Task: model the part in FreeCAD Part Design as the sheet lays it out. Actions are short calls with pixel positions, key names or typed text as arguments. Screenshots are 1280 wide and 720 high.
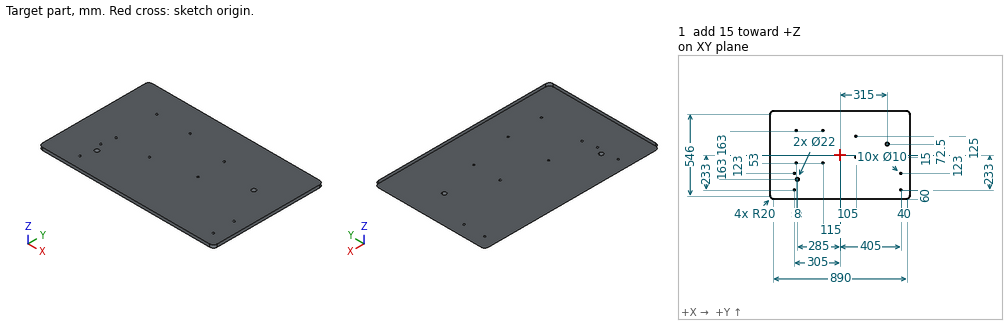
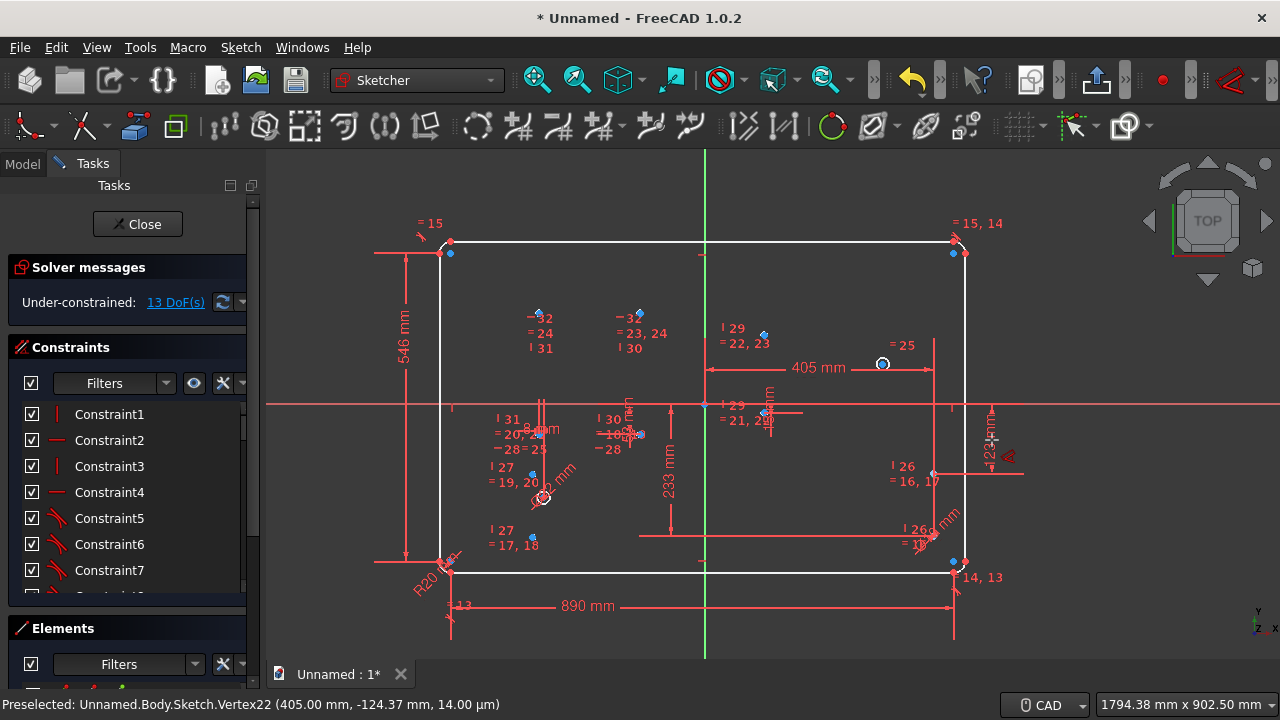
click(533, 537)
click(619, 370)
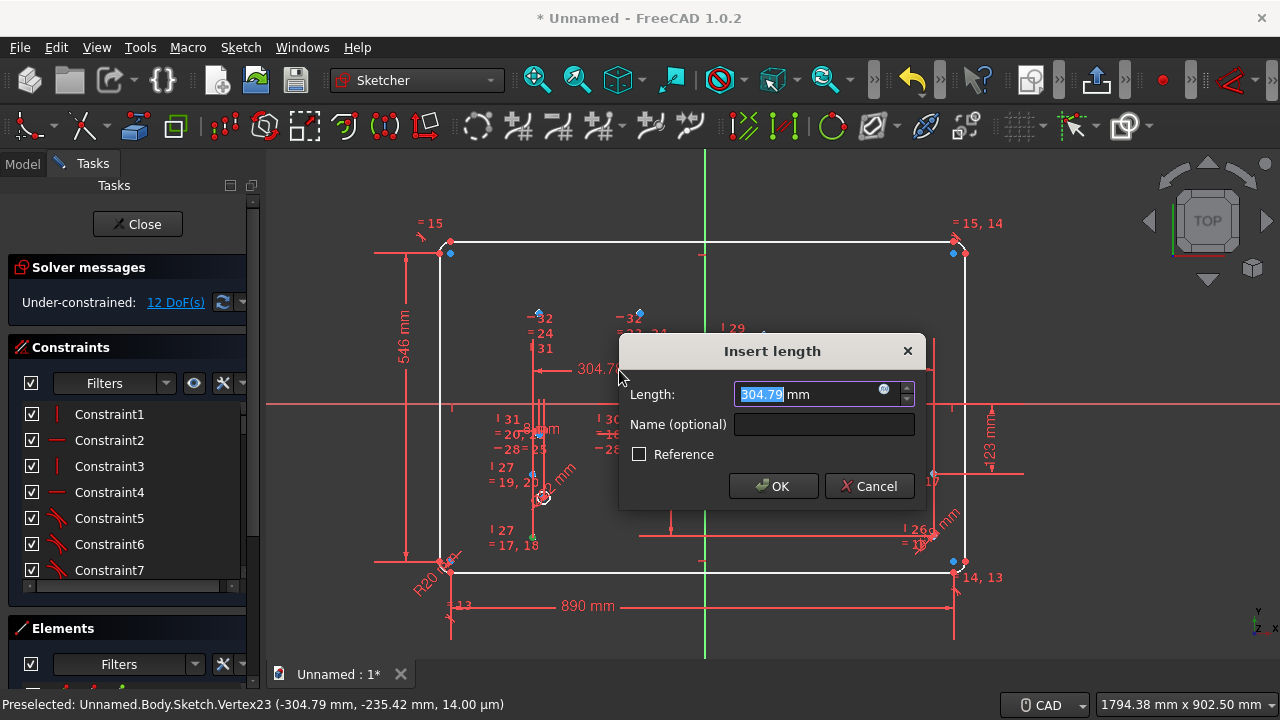
text(305)
key(Return)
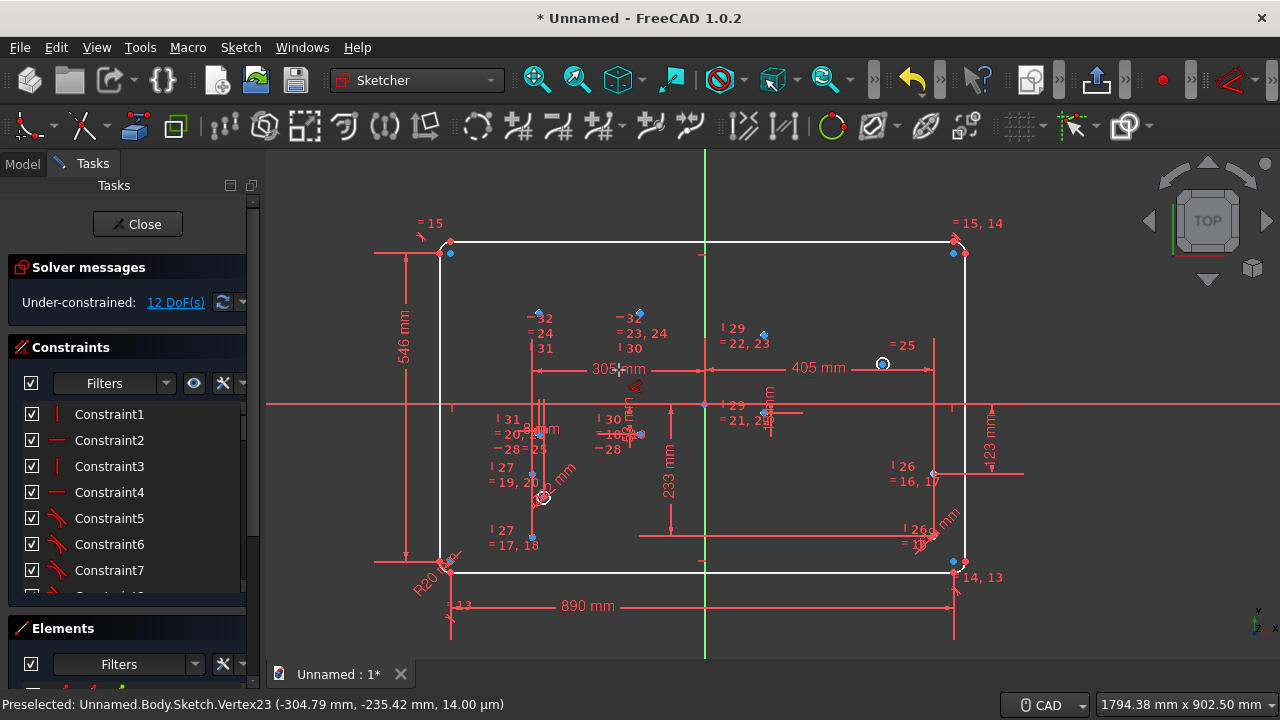
click(532, 537)
click(498, 518)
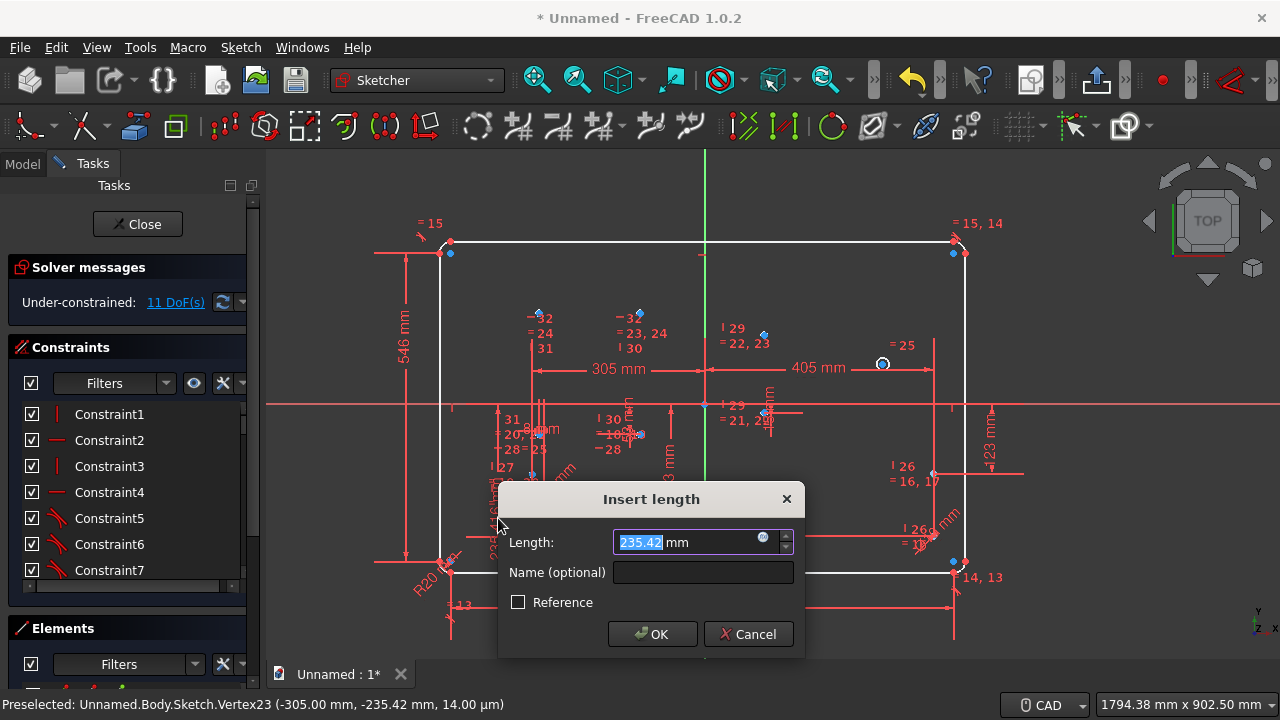
text(233)
key(Return)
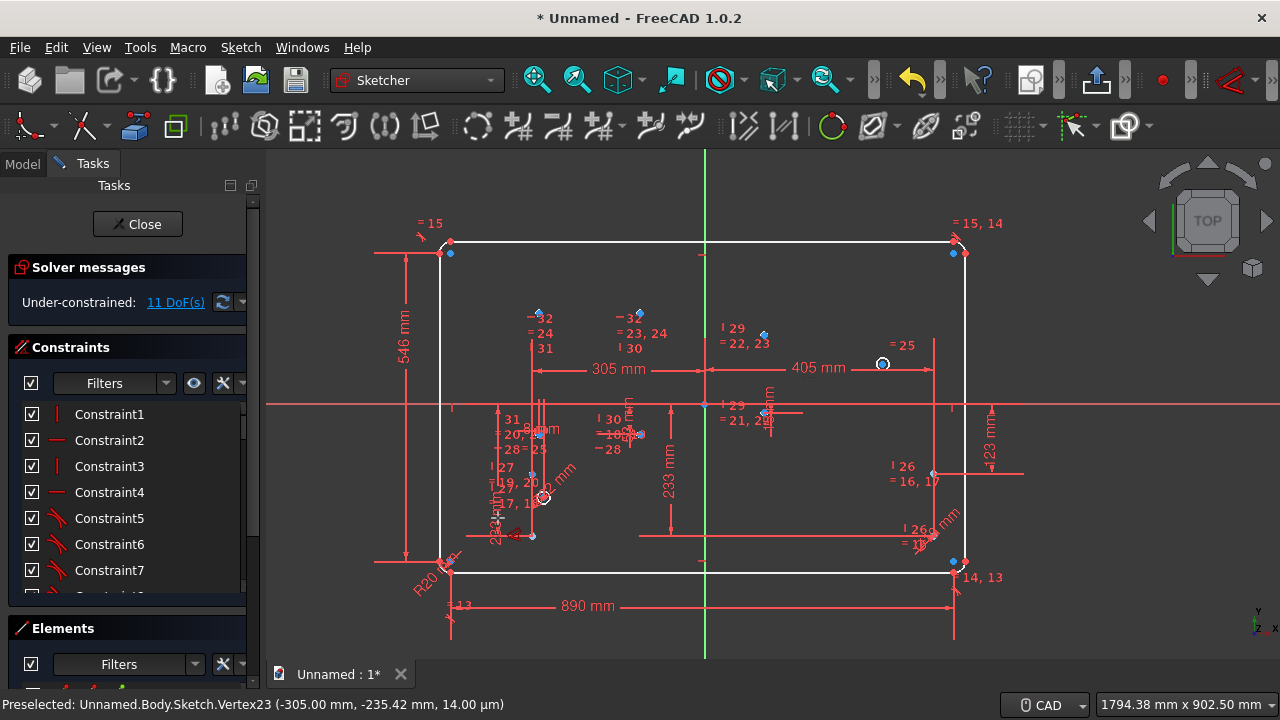
click(544, 498)
click(624, 532)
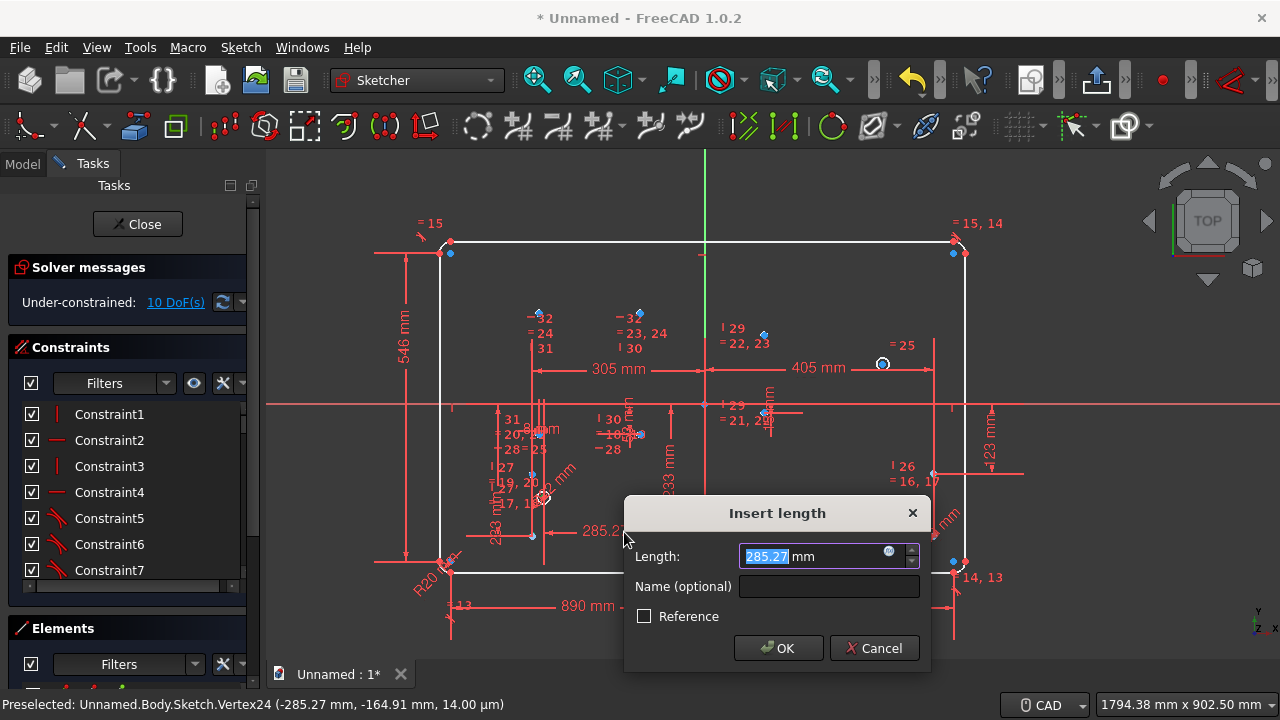
text(285)
key(Return)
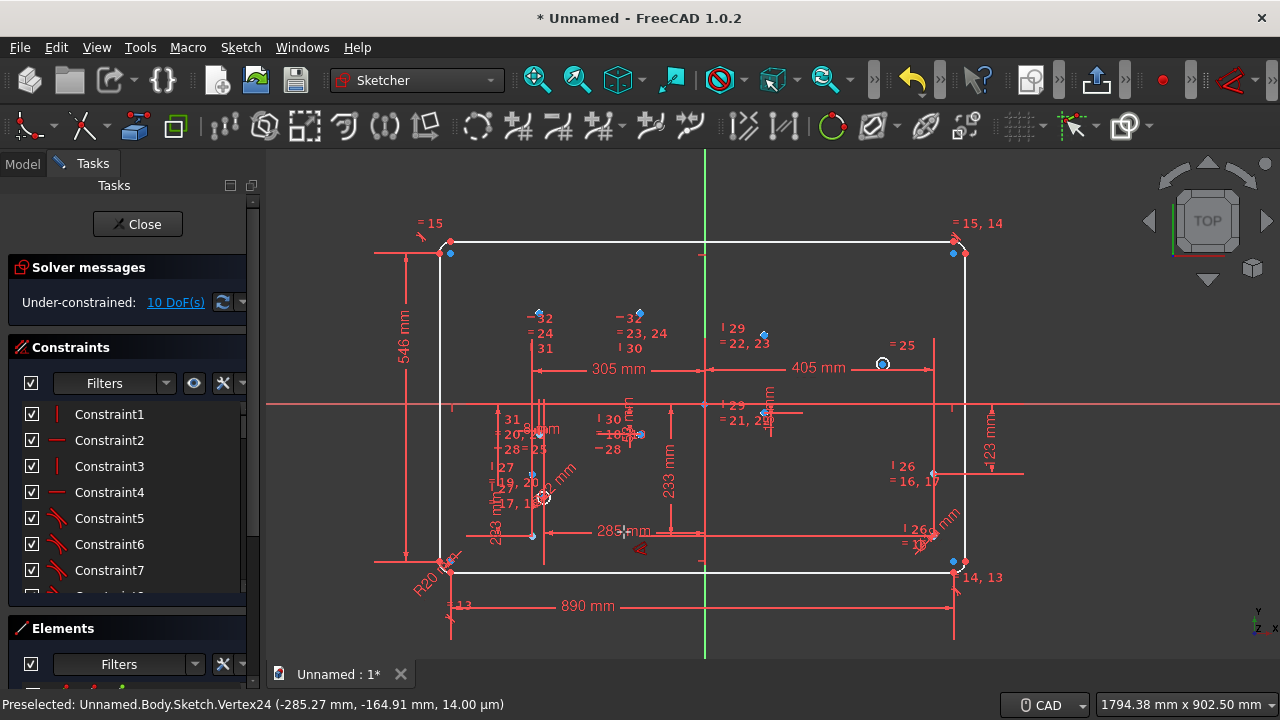
click(544, 498)
click(510, 451)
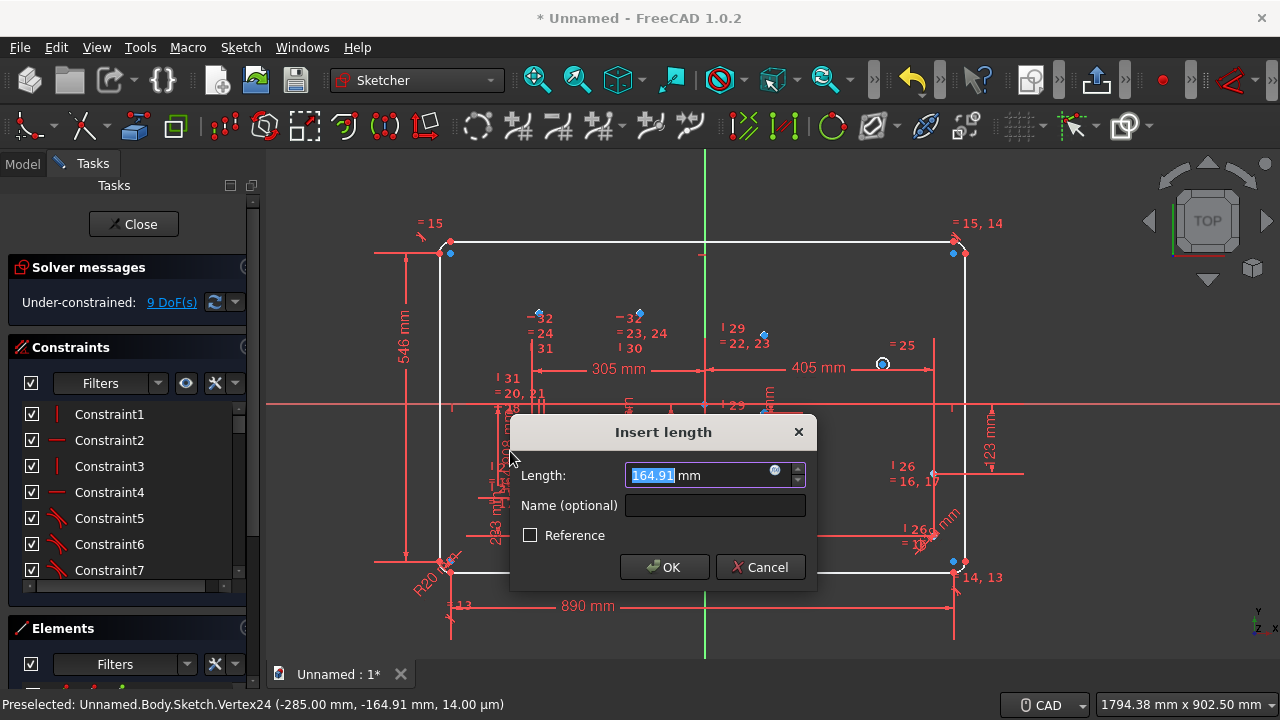
text(163)
key(Return)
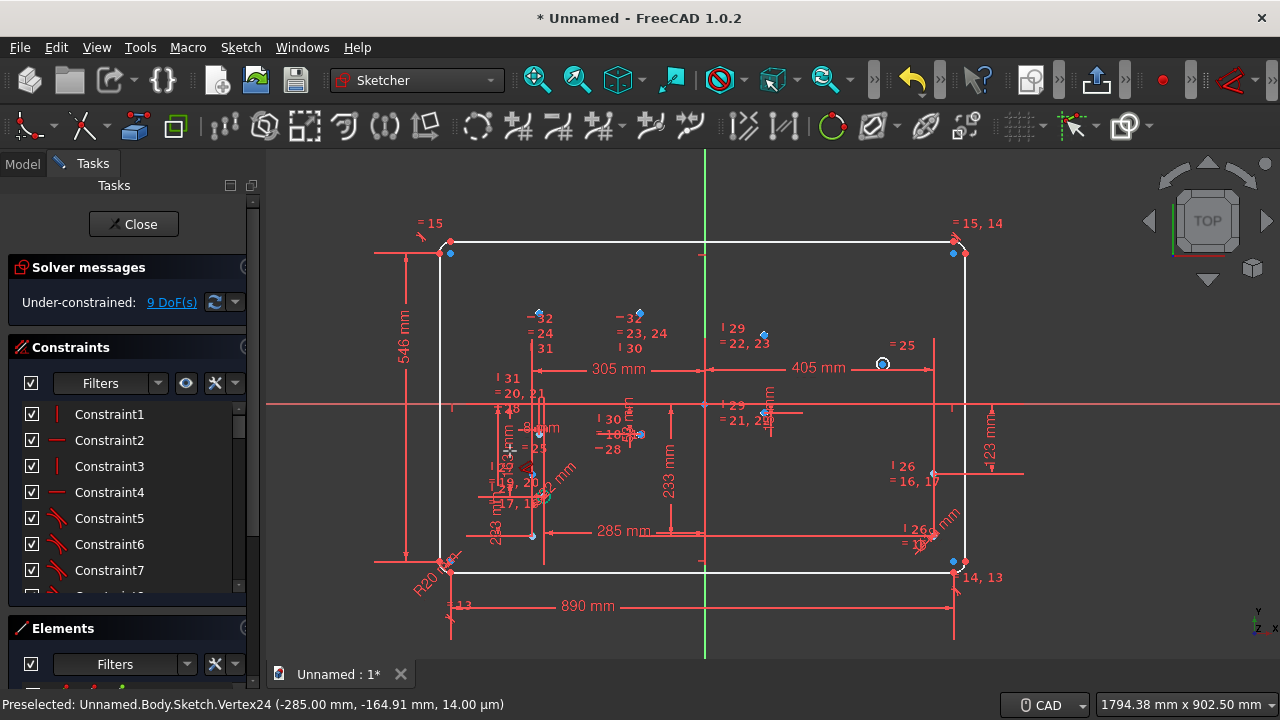
click(640, 434)
click(672, 492)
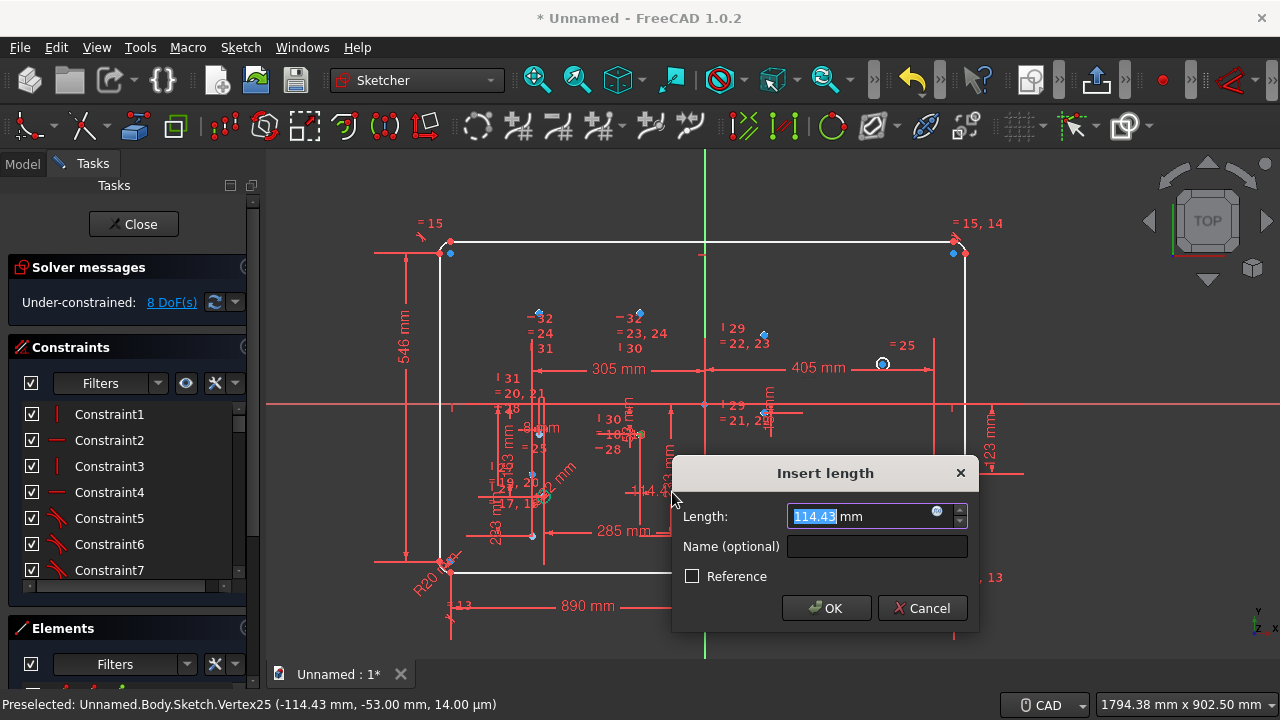
text(115)
key(Return)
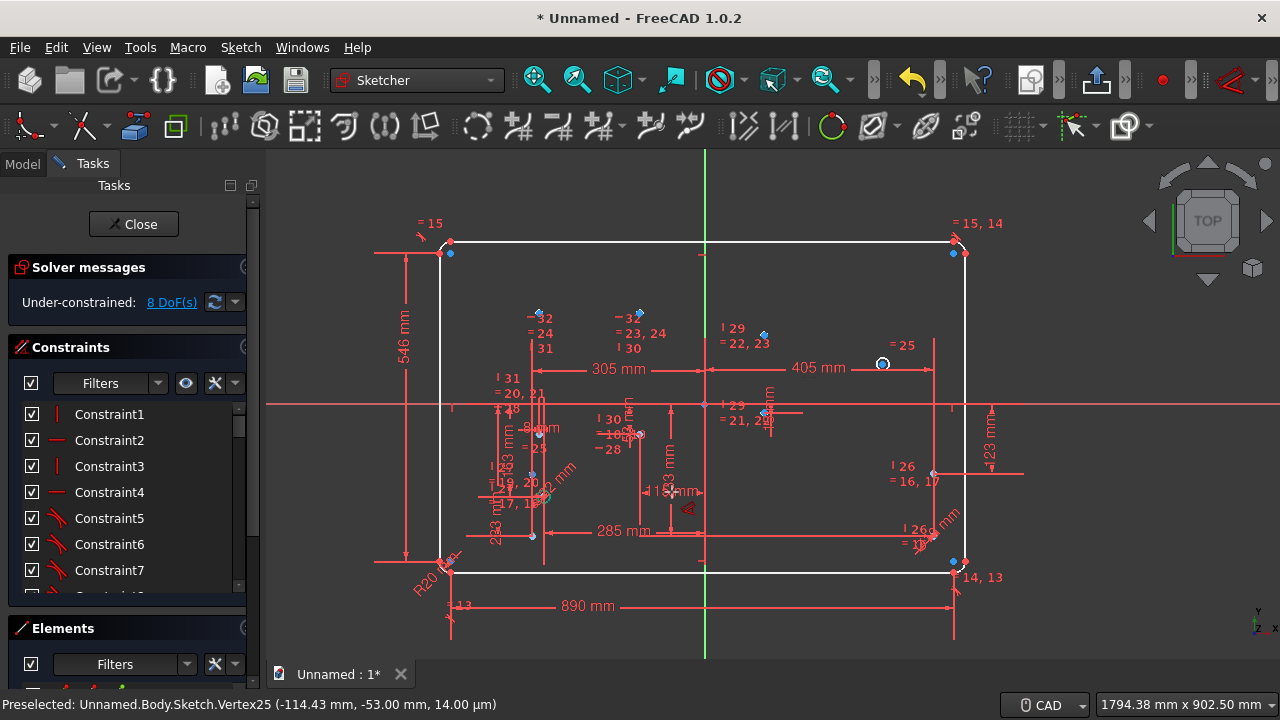
click(532, 475)
click(739, 439)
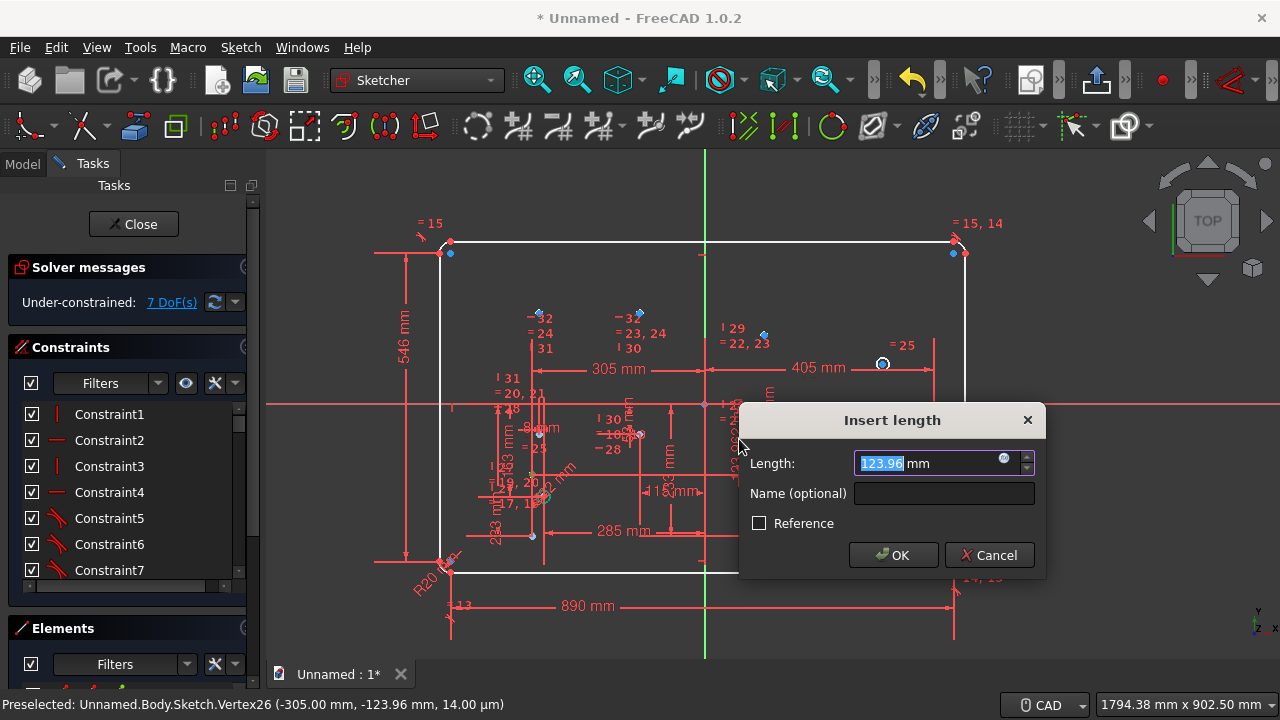
text(123)
key(Return)